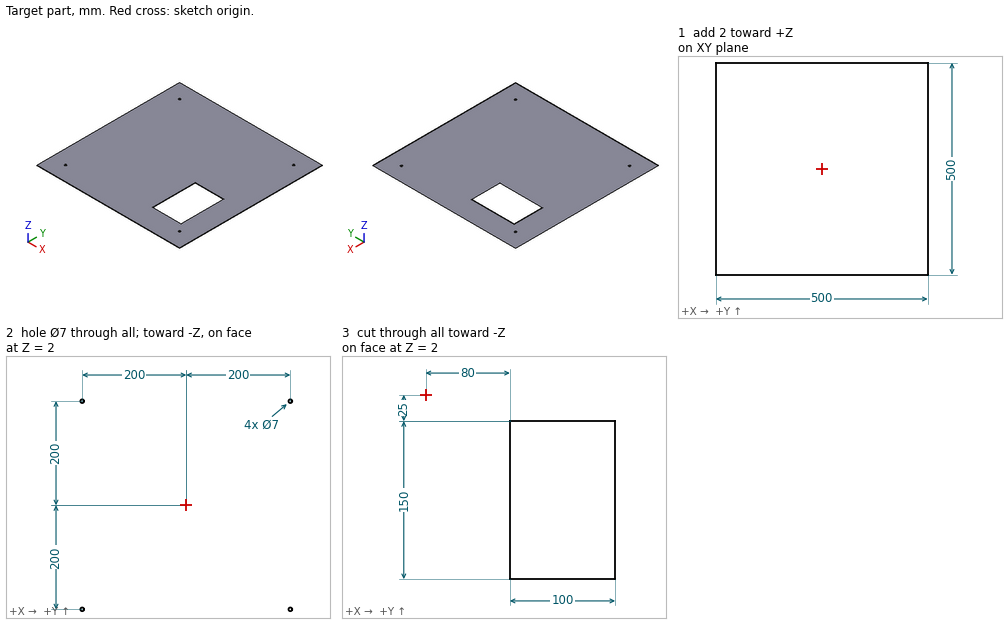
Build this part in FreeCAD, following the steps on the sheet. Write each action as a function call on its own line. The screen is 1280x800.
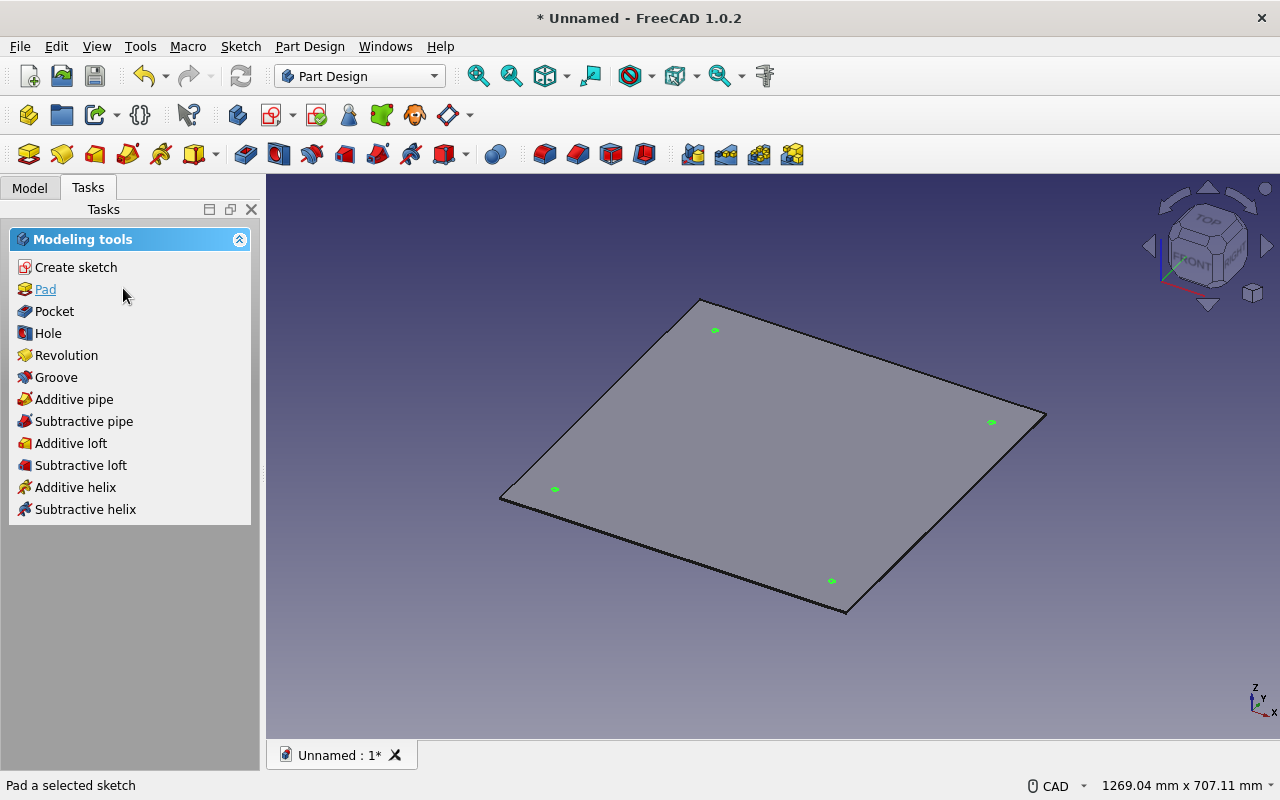
click(279, 154)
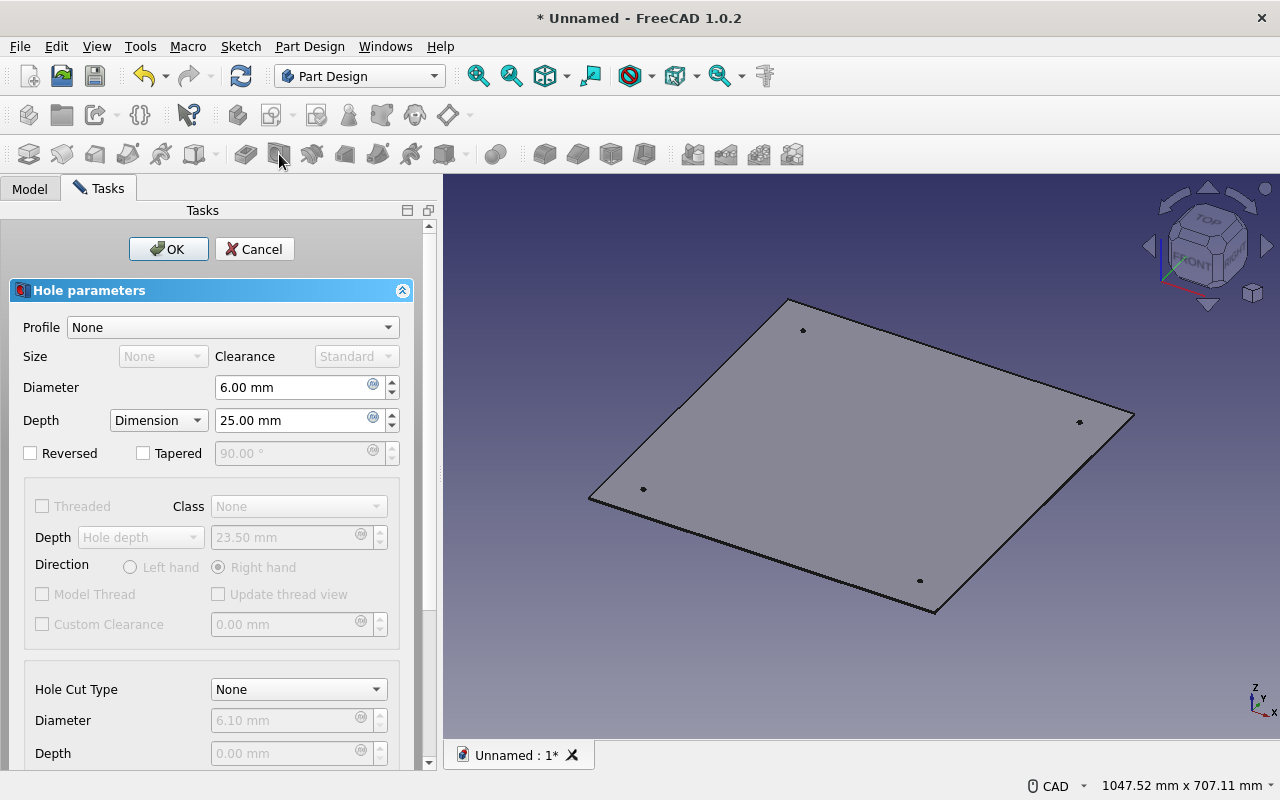
triple_click(300, 388)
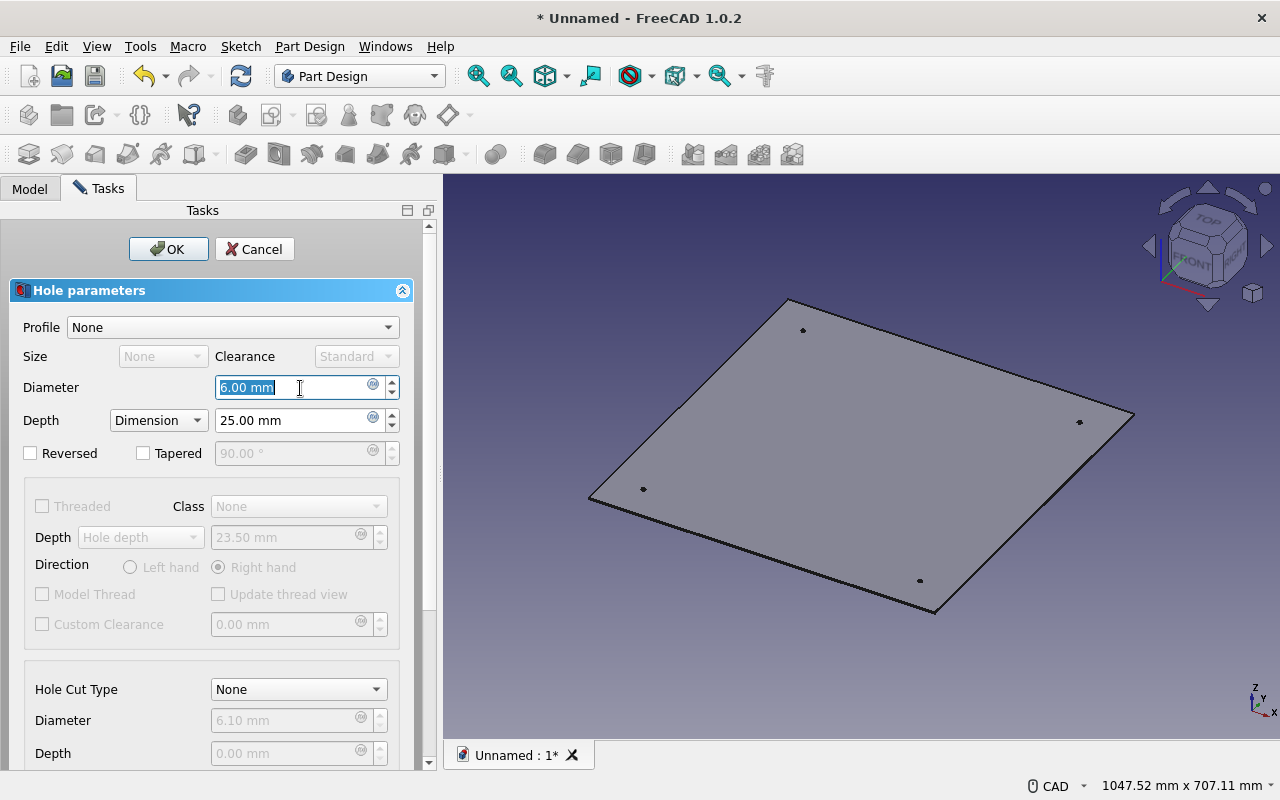
text(7)
key(Tab)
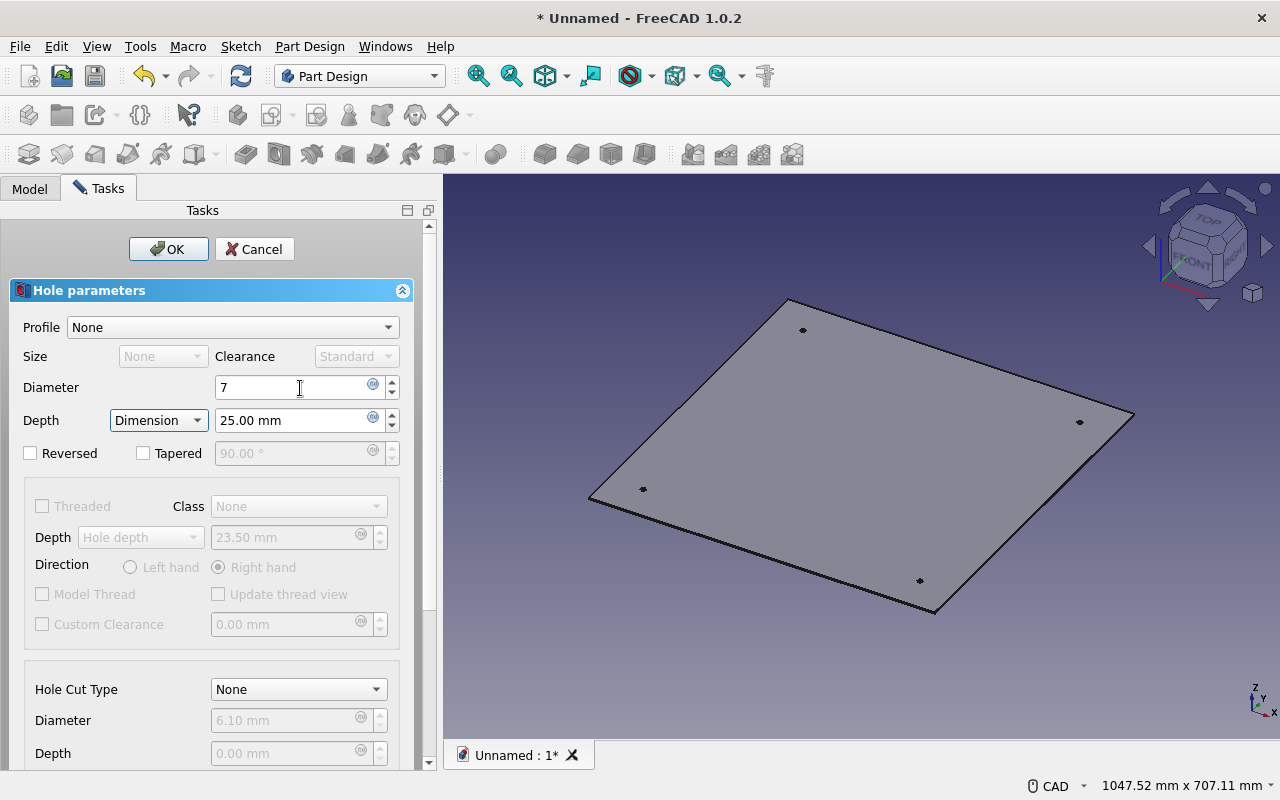
click(160, 420)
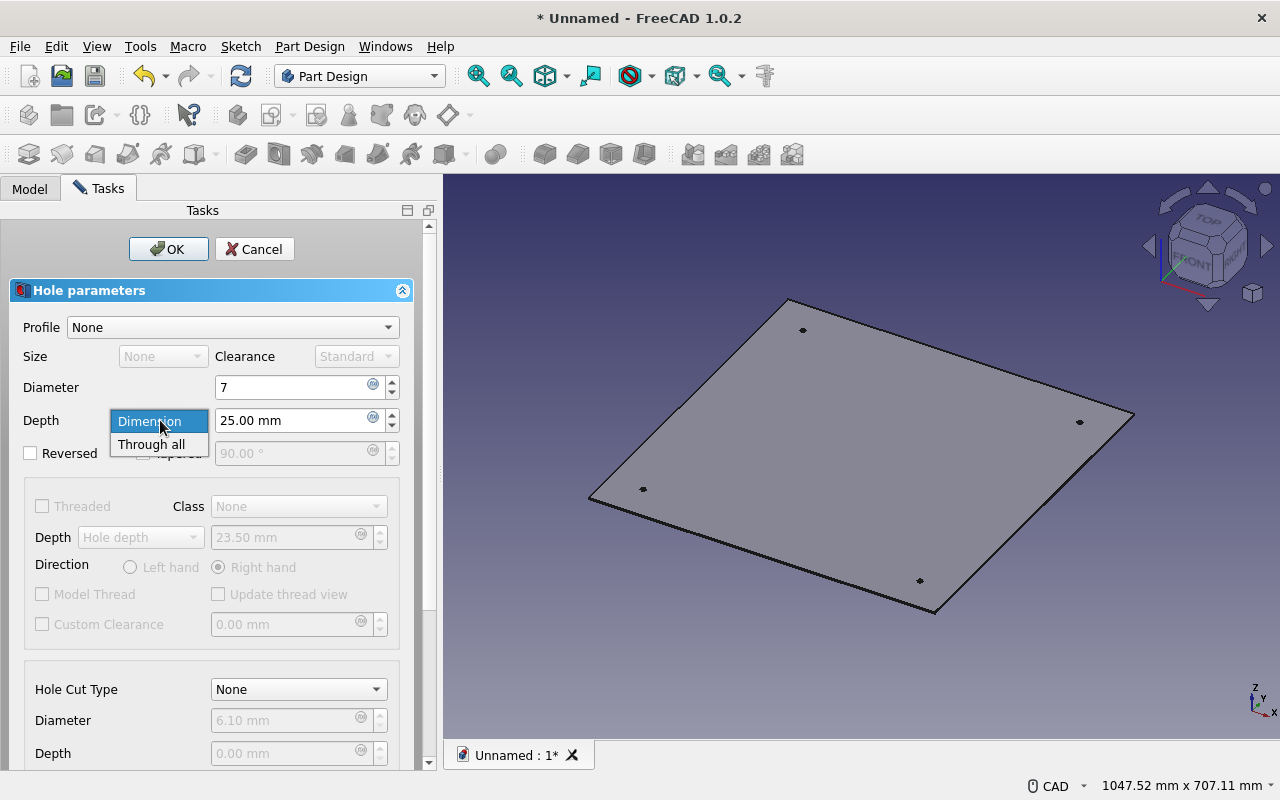
click(158, 444)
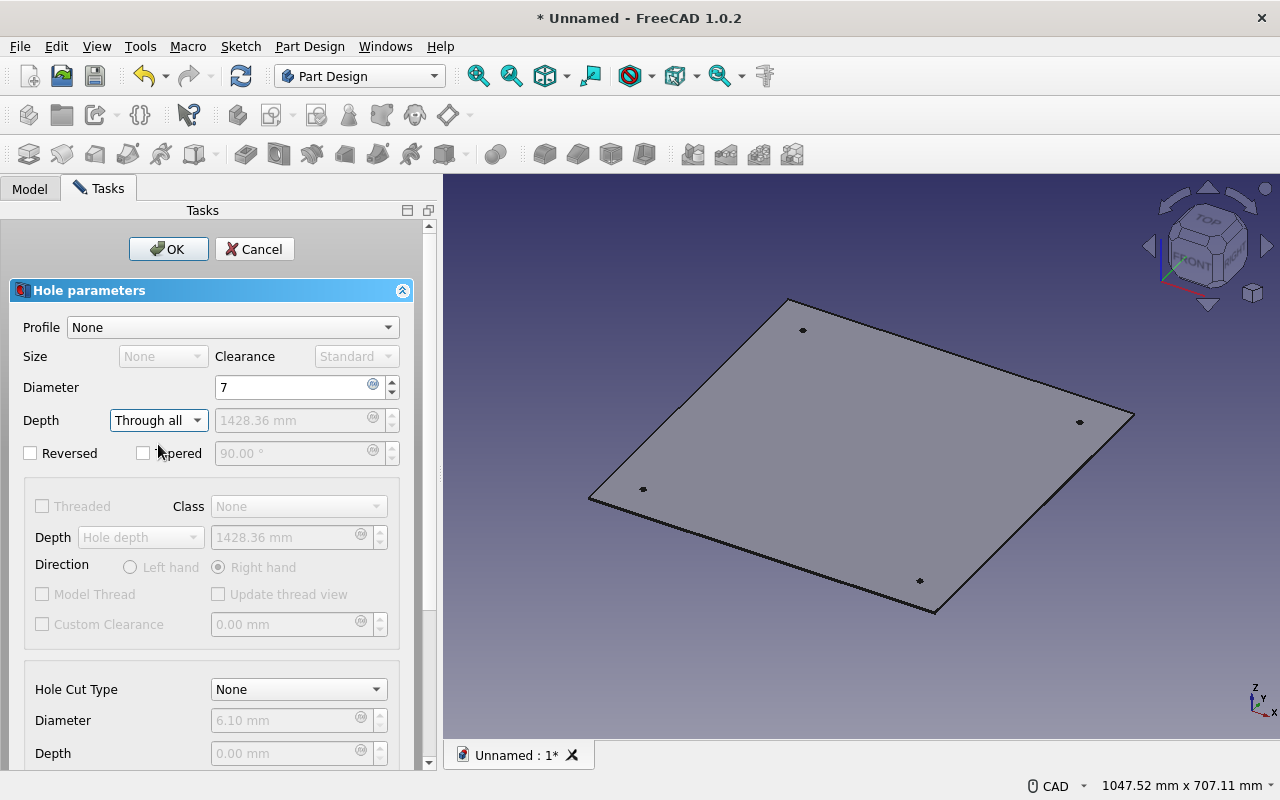
click(169, 249)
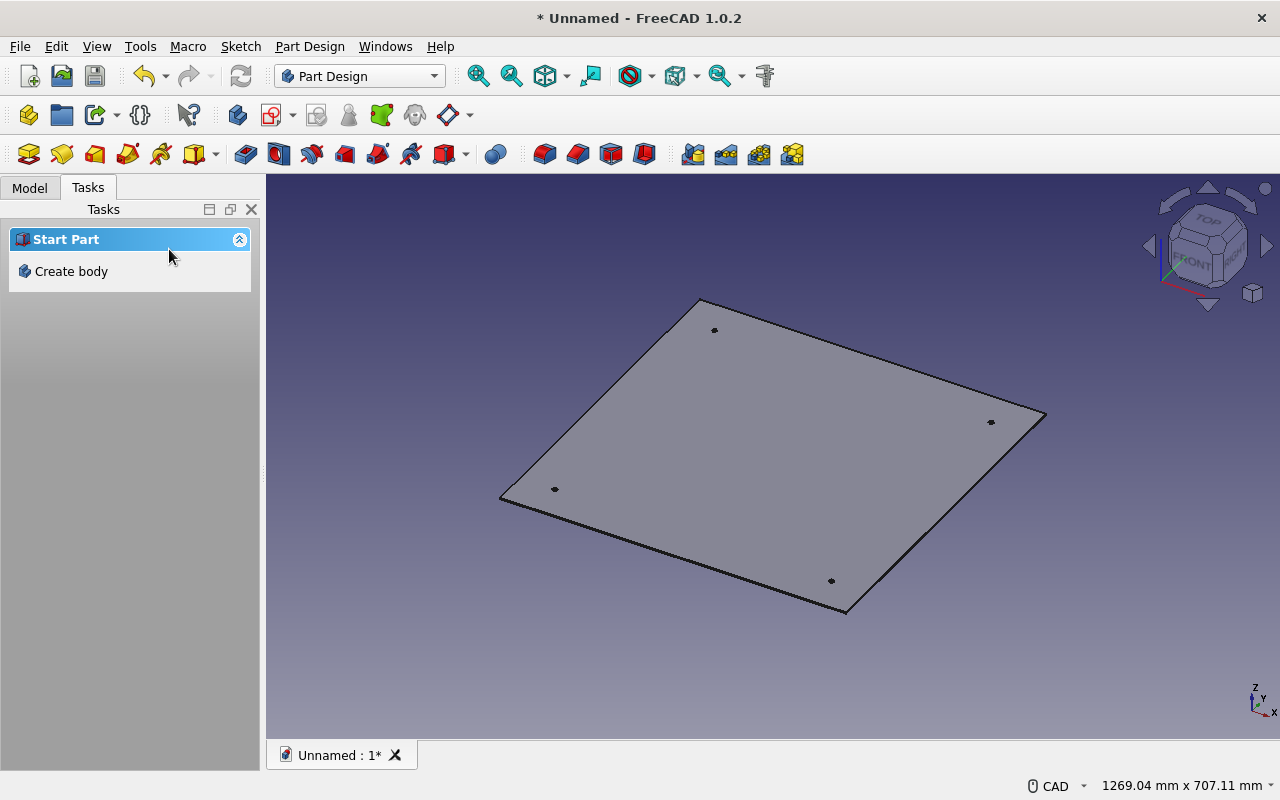
click(773, 455)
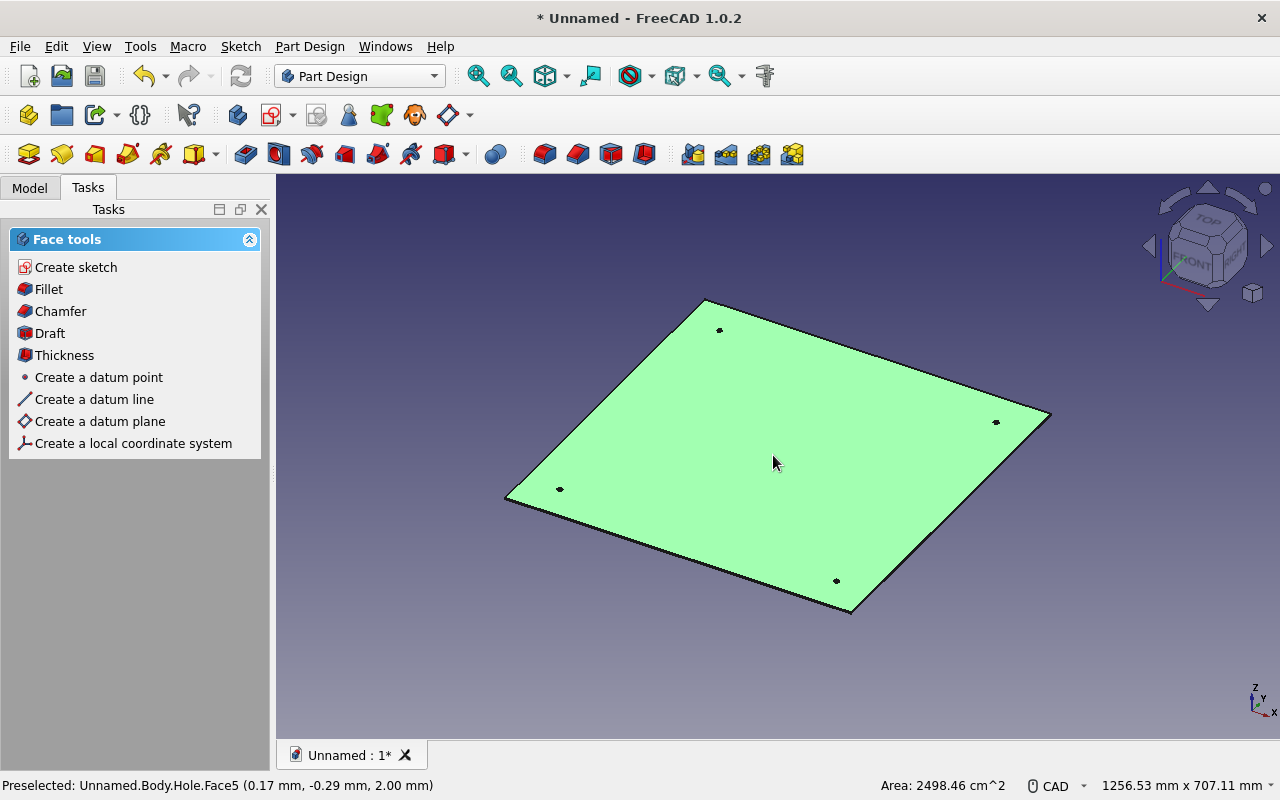
click(270, 116)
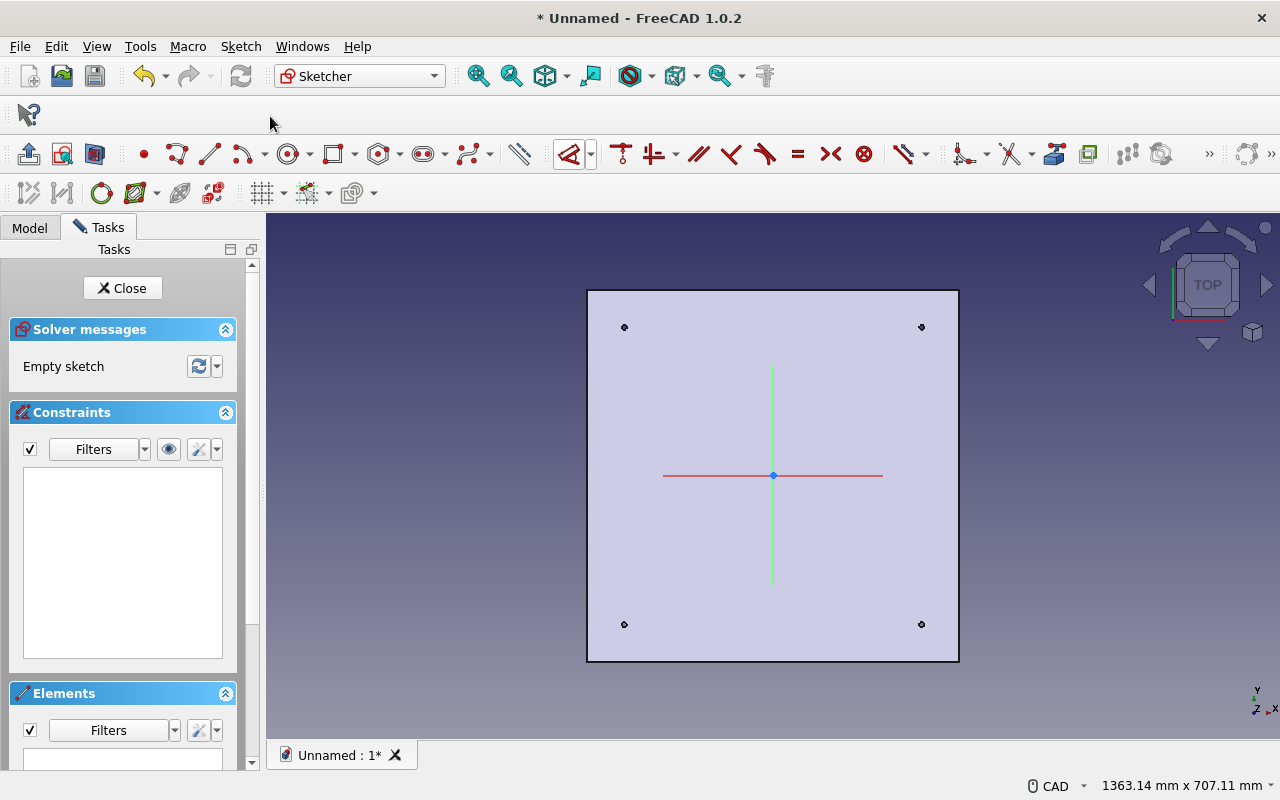
scroll(919, 579, up, 5)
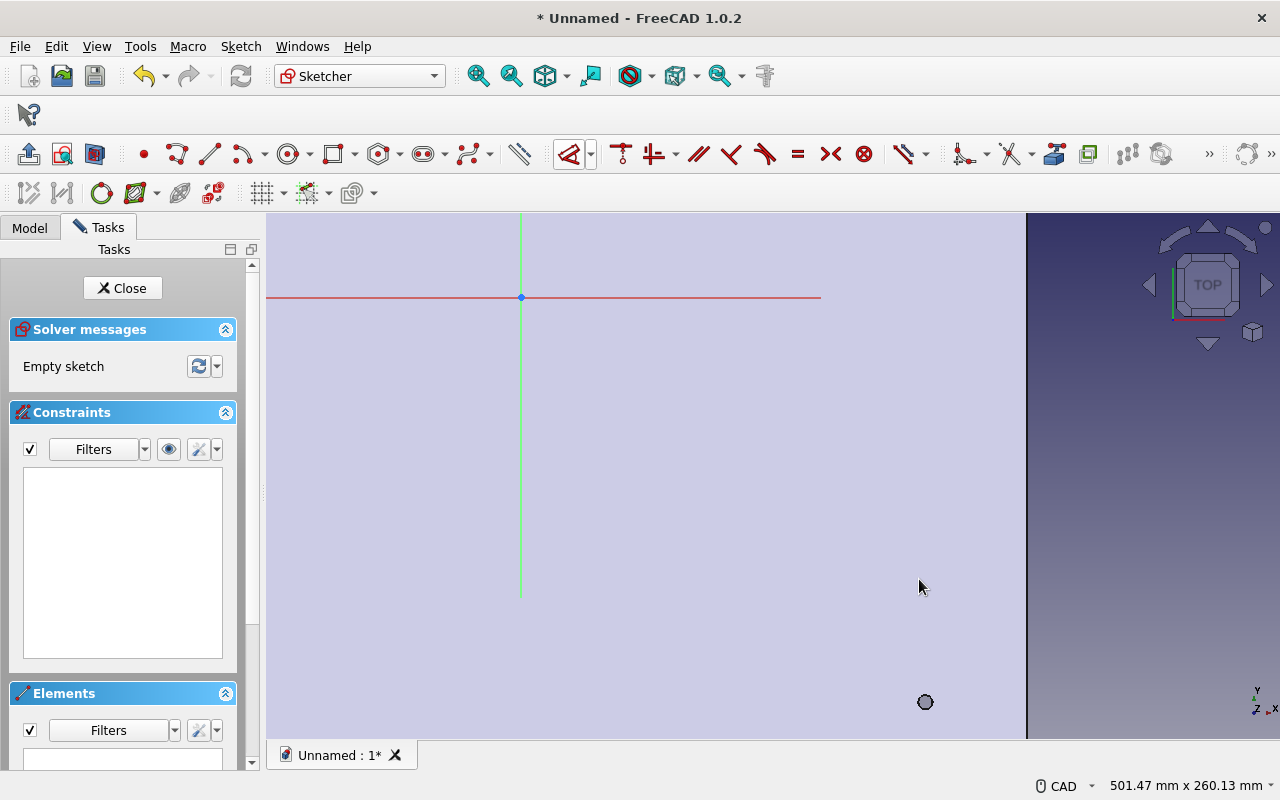
key(g)
key(r)